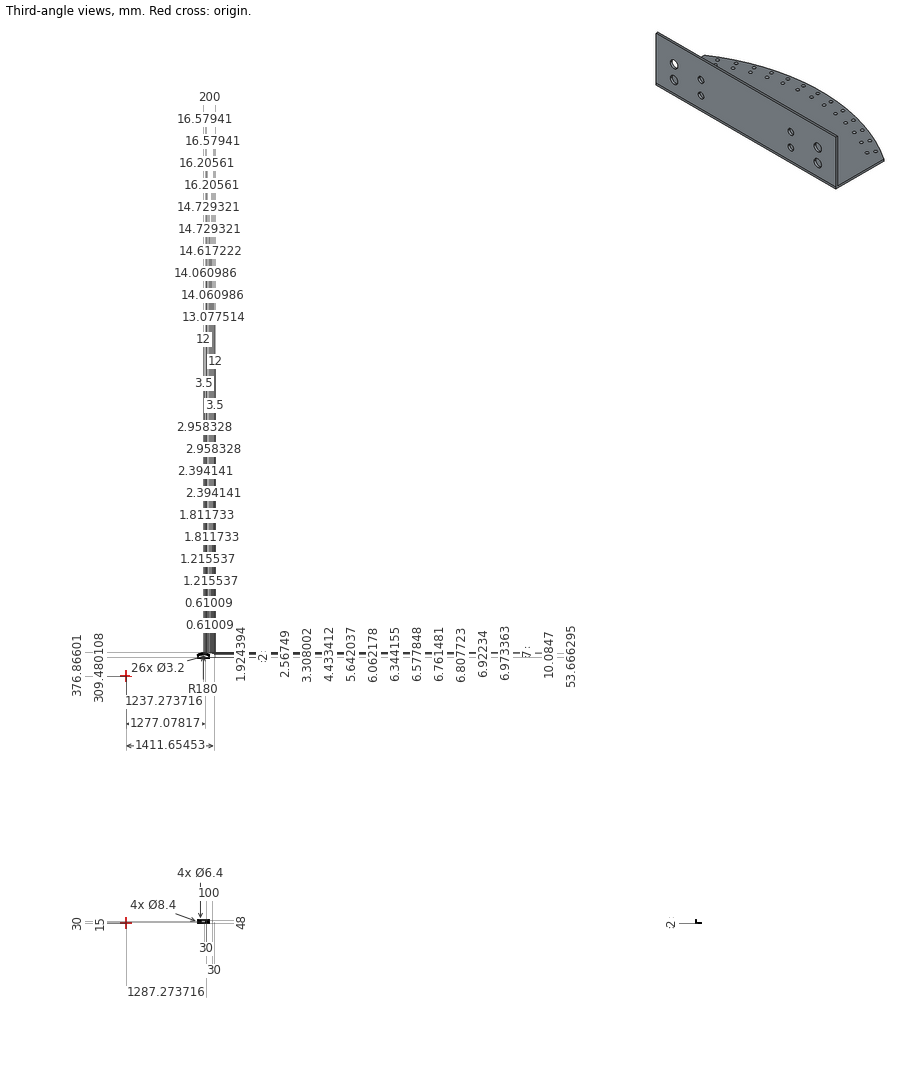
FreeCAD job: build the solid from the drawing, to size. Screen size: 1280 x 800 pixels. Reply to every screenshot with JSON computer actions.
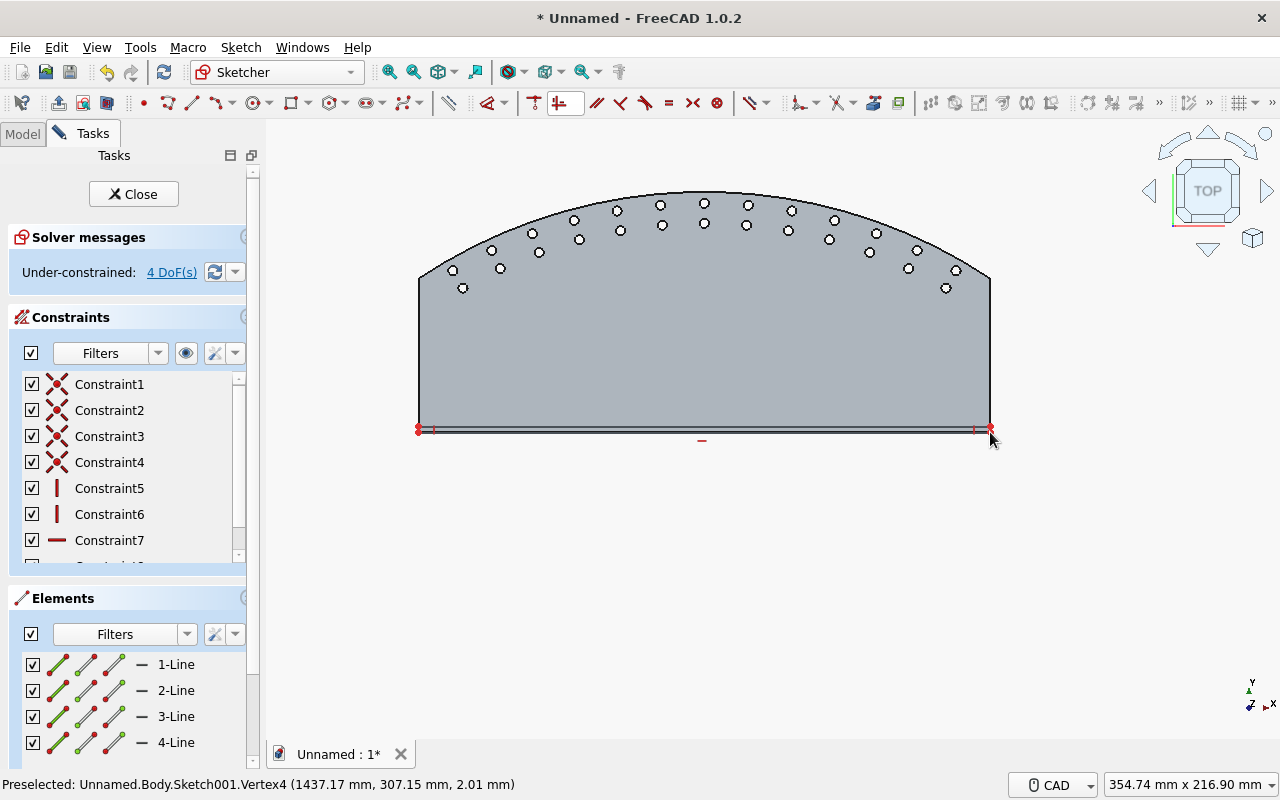
{"action": "key", "text": "d"}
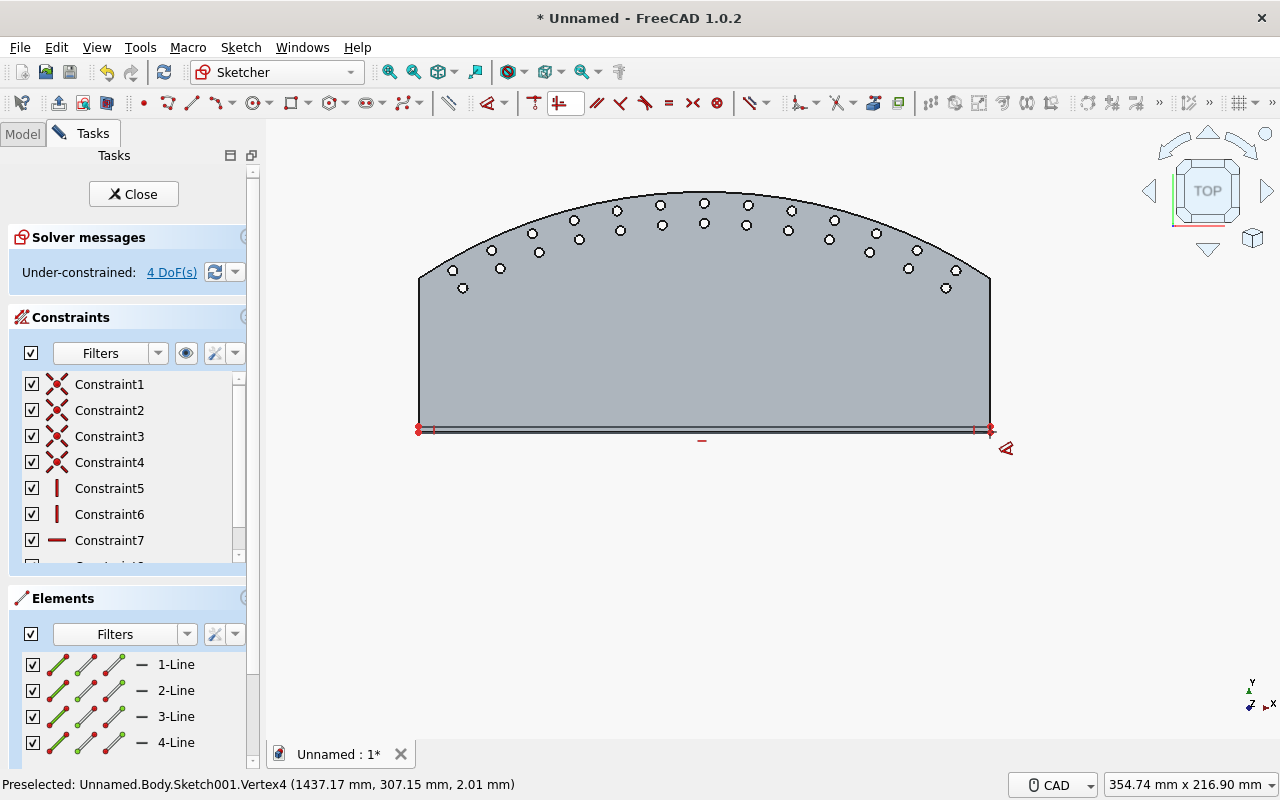
{"action": "scroll", "coordinate": [419, 430], "scroll_direction": "up", "scroll_amount": 10}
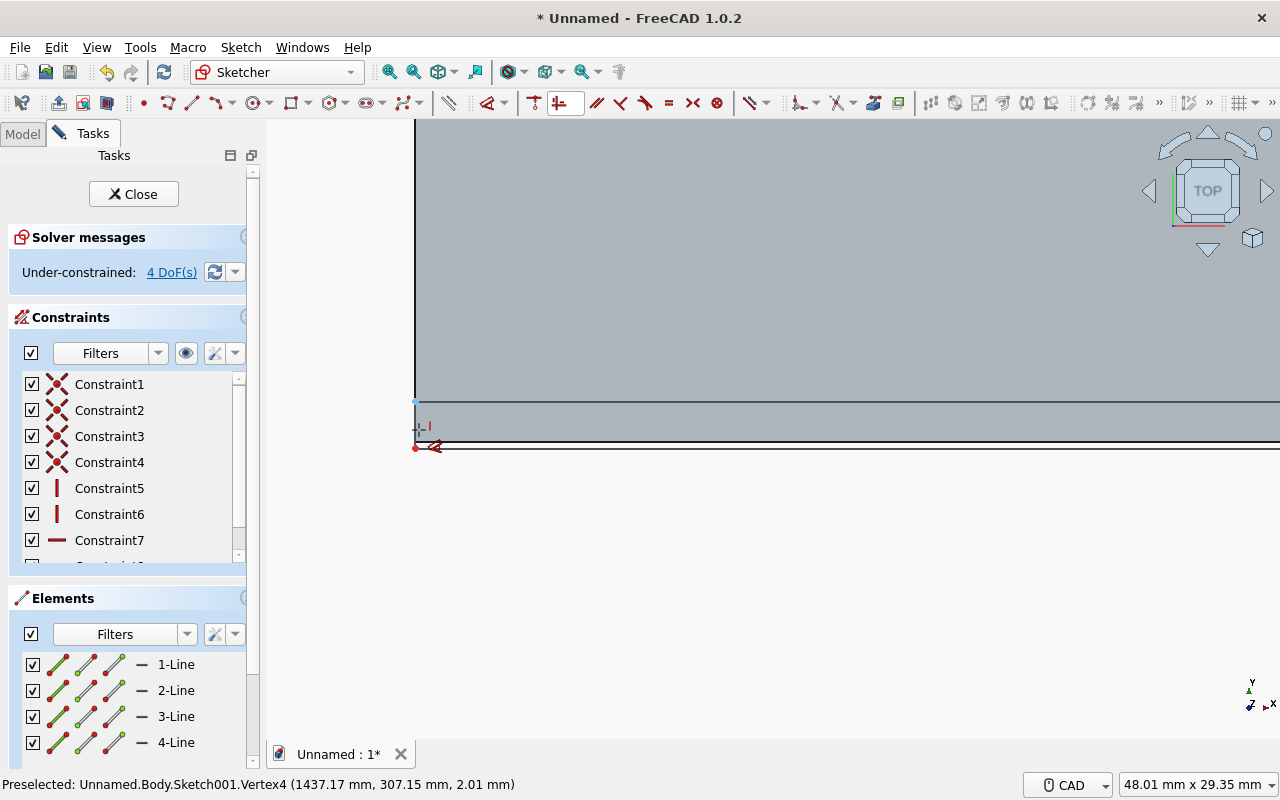
{"action": "left_click", "coordinate": [415, 425]}
{"action": "left_click", "coordinate": [381, 425]}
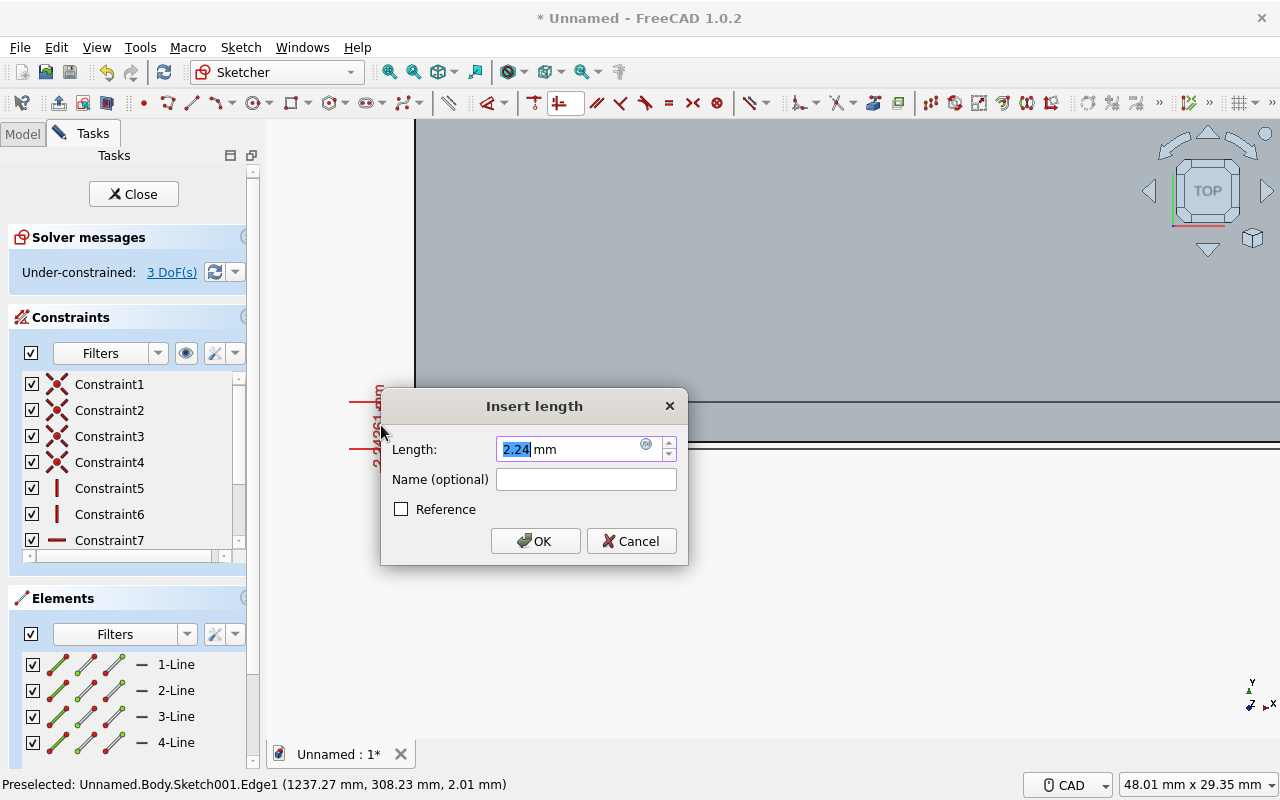
{"action": "type", "text": "2"}
{"action": "key", "text": "Return"}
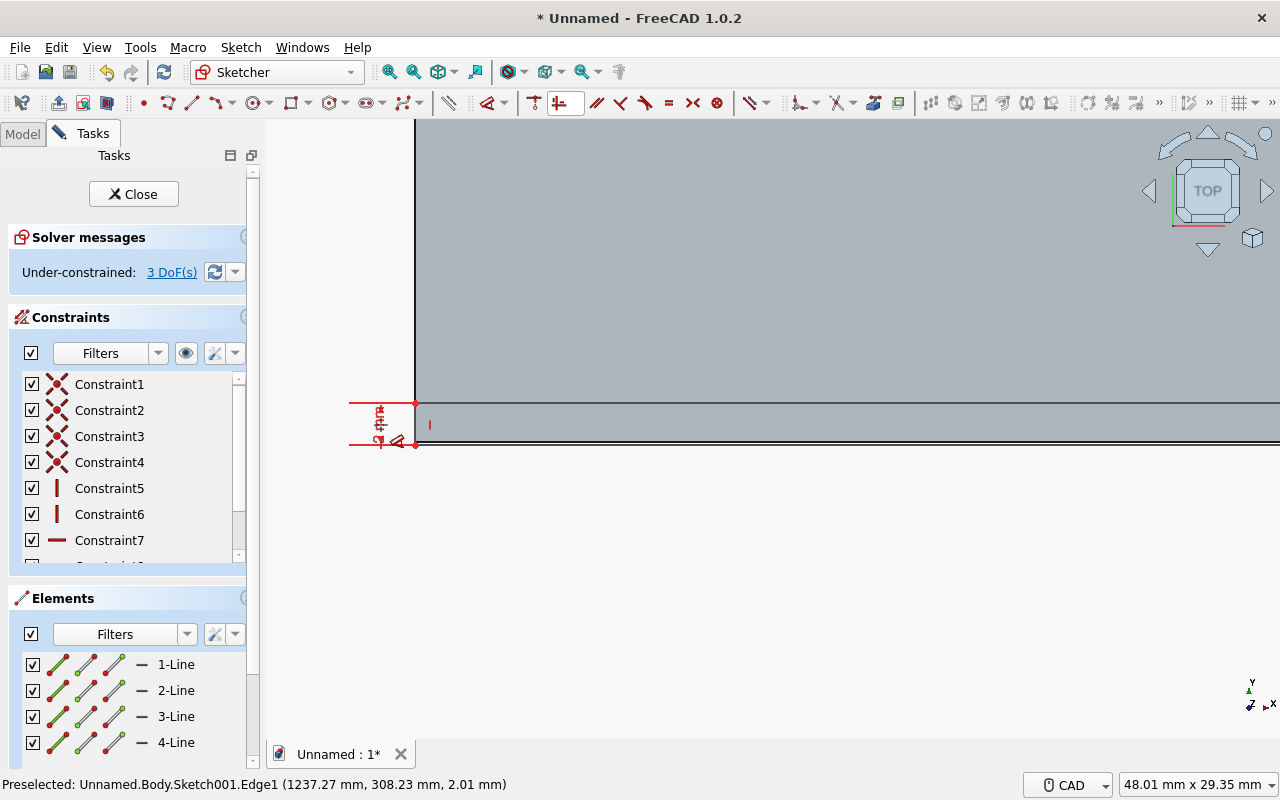
{"action": "scroll", "coordinate": [419, 430], "scroll_direction": "down", "scroll_amount": 10}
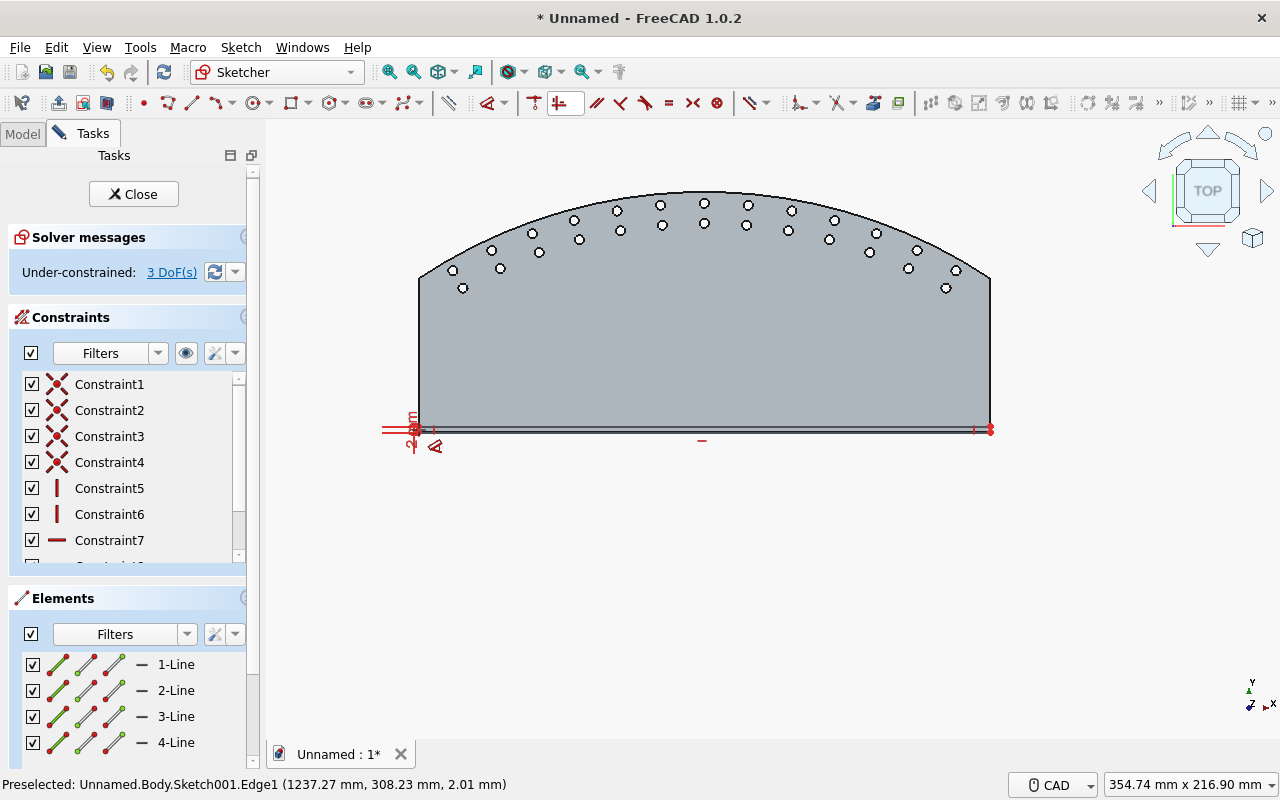
{"action": "scroll", "coordinate": [590, 433], "scroll_direction": "up", "scroll_amount": 5}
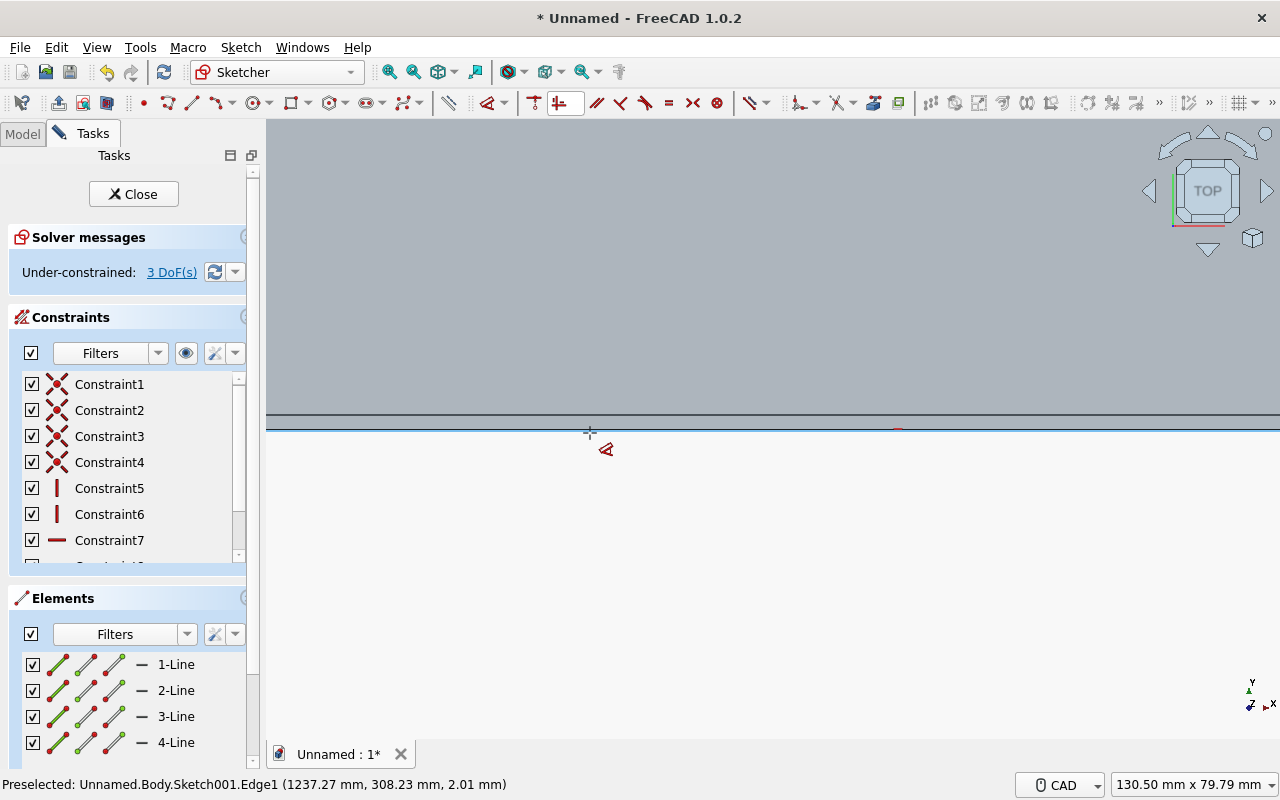
{"action": "left_click", "coordinate": [590, 431]}
{"action": "left_click", "coordinate": [704, 465]}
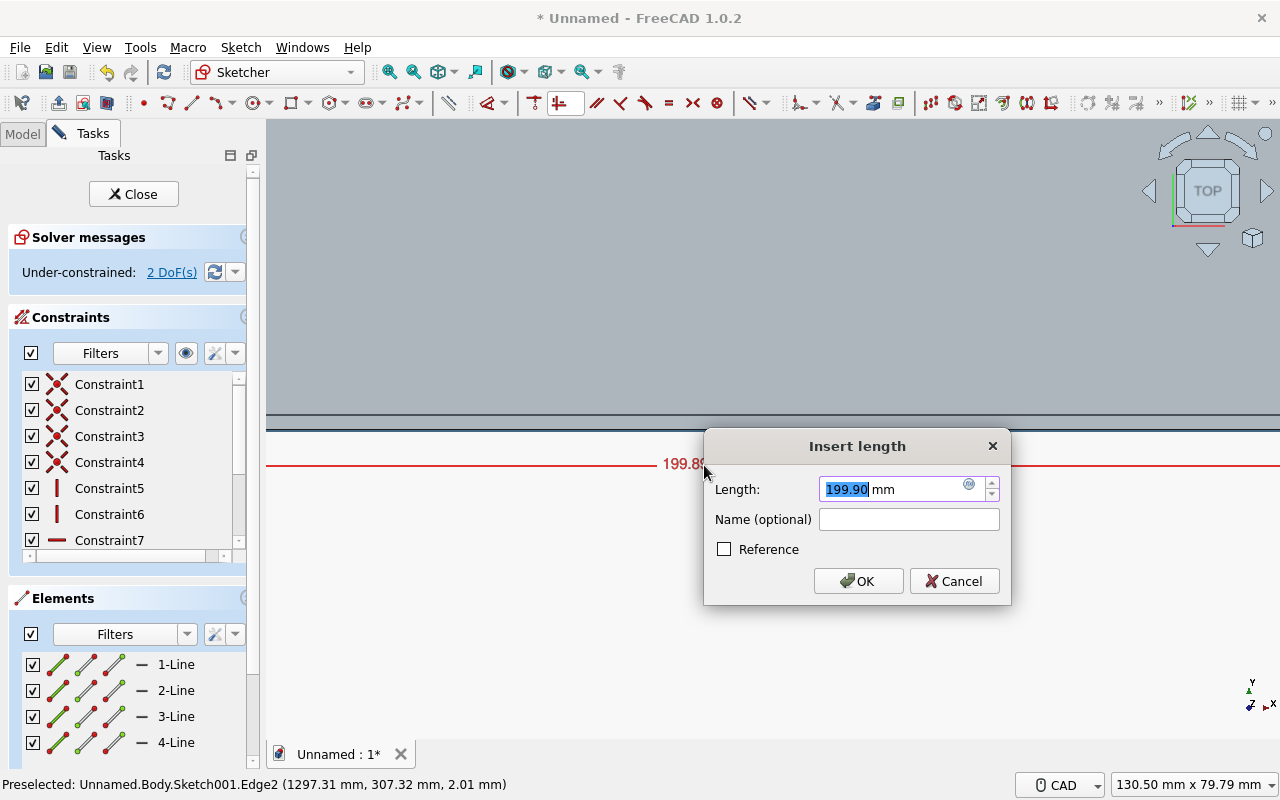
{"action": "type", "text": "200"}
{"action": "key", "text": "Return"}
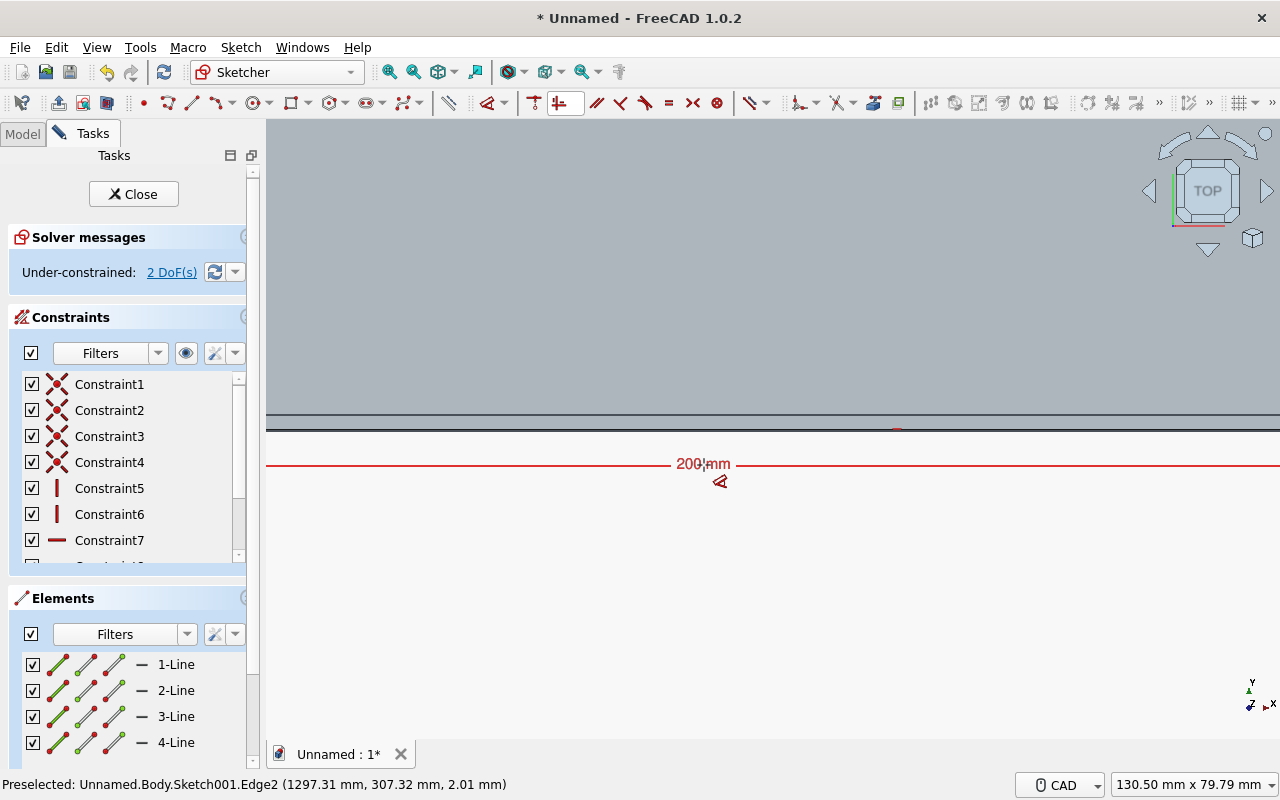
{"action": "scroll", "coordinate": [590, 433], "scroll_direction": "down", "scroll_amount": 5}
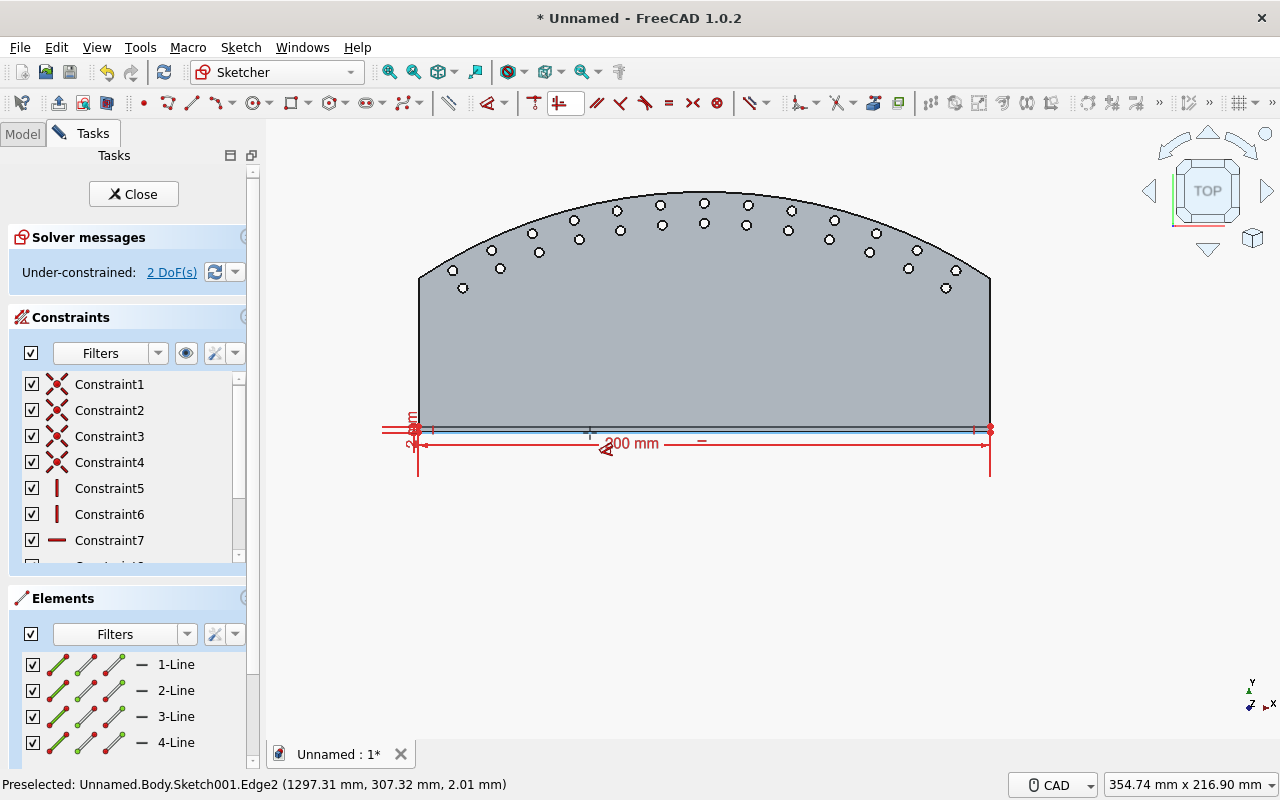
{"action": "scroll", "coordinate": [418, 427], "scroll_direction": "up", "scroll_amount": 4}